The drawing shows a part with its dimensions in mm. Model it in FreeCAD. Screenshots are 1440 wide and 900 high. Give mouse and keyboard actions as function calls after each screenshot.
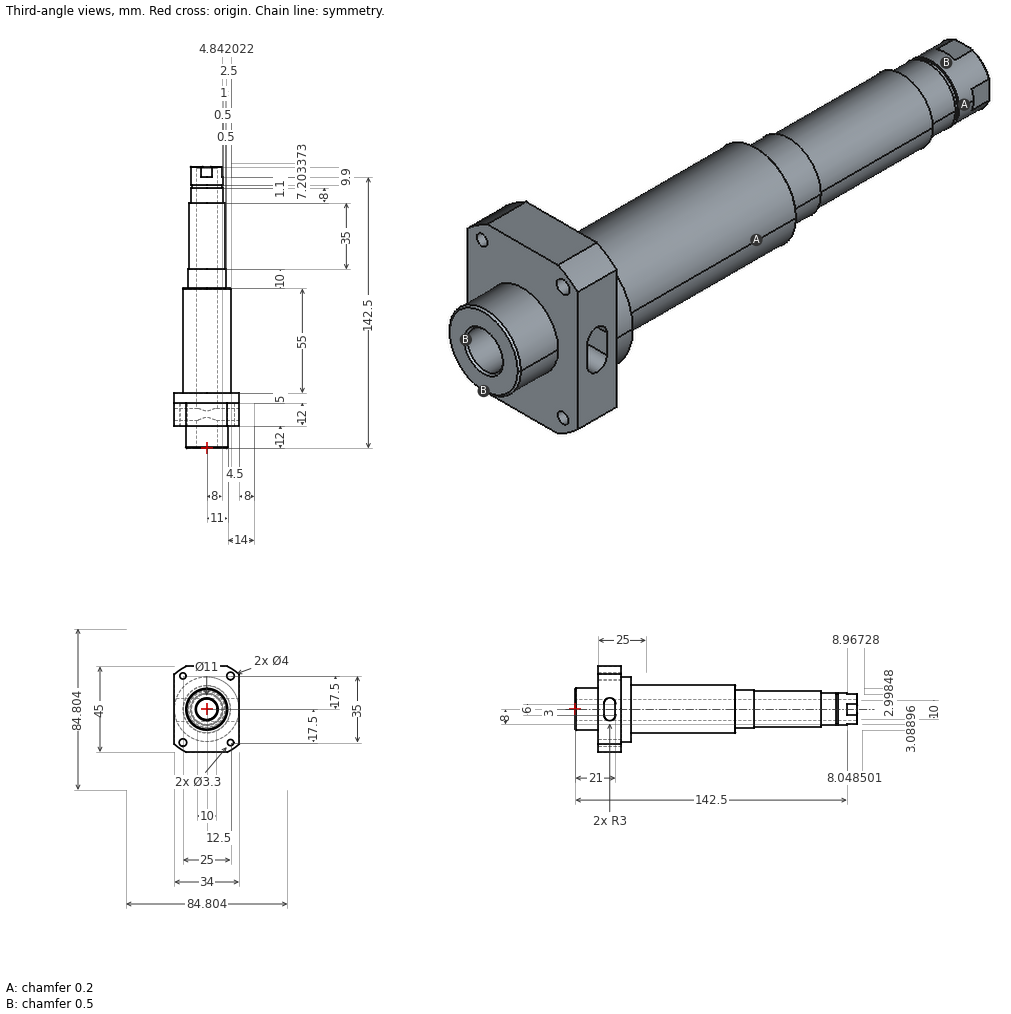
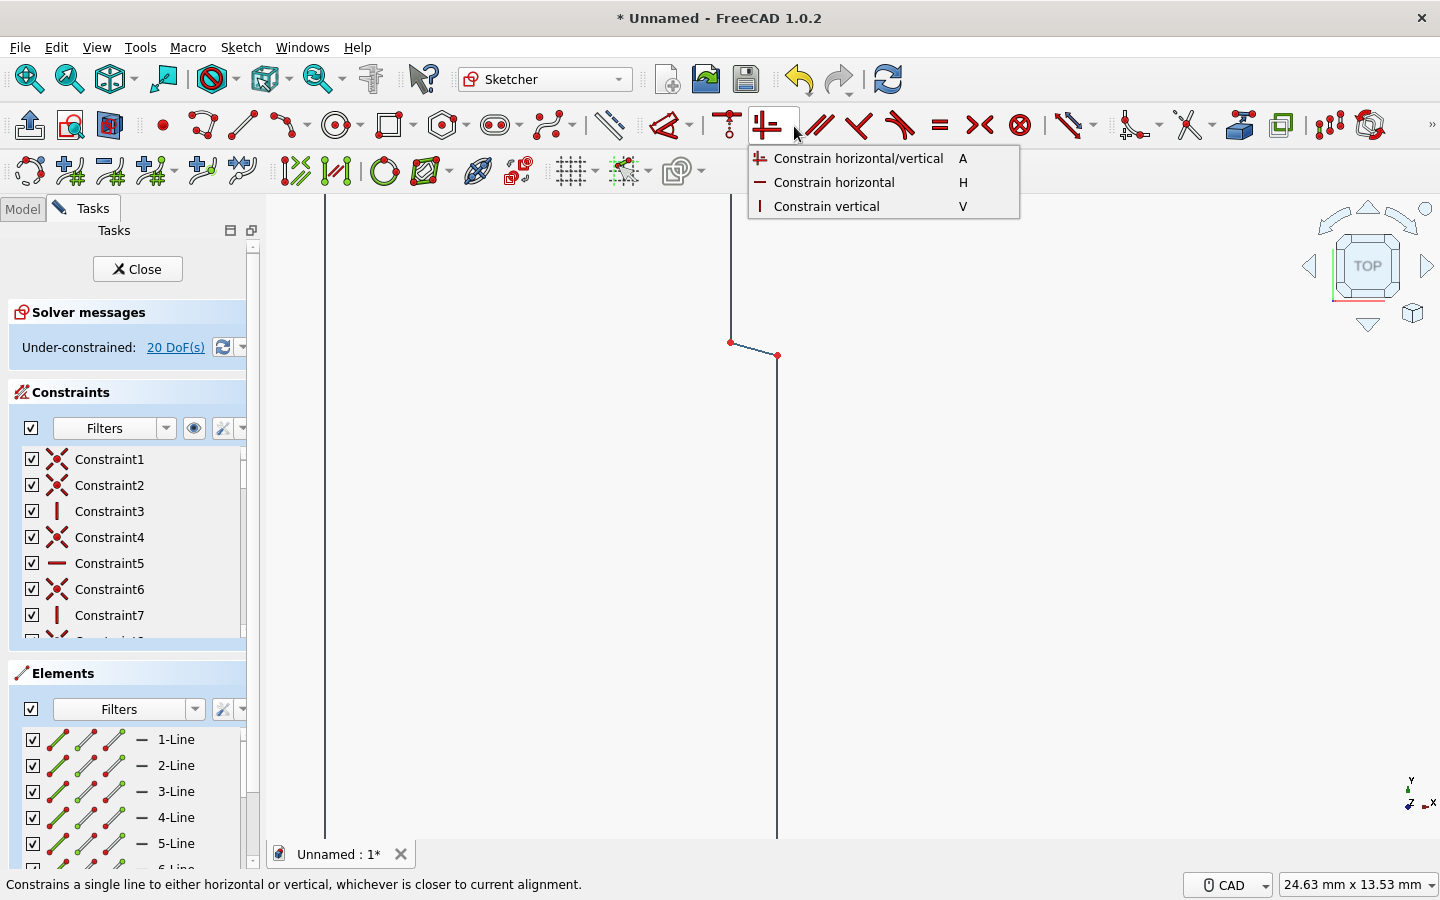
click(884, 182)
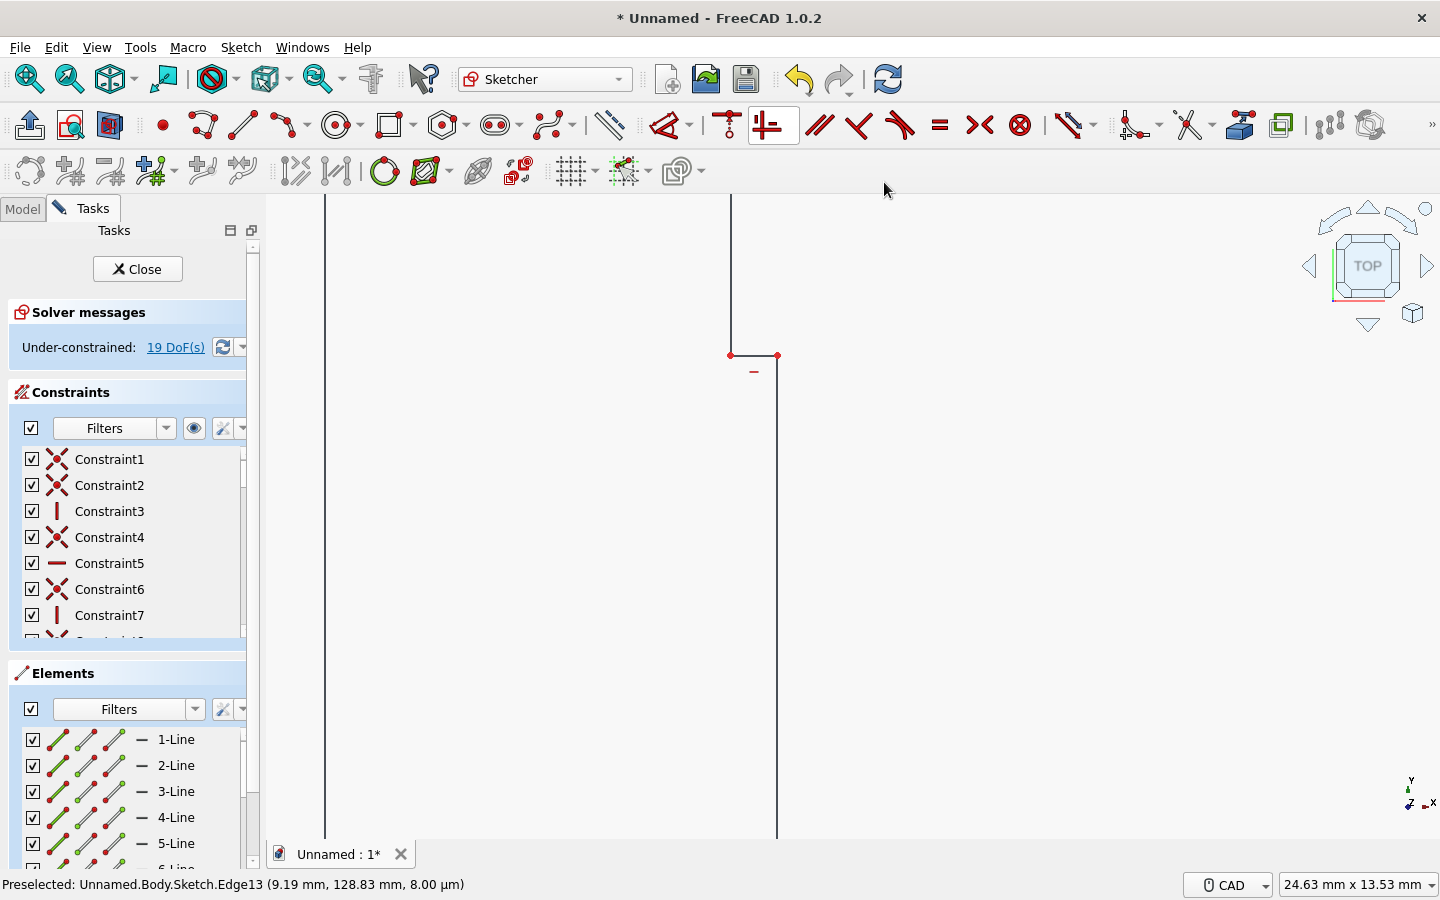
scroll(776, 358, down, 14)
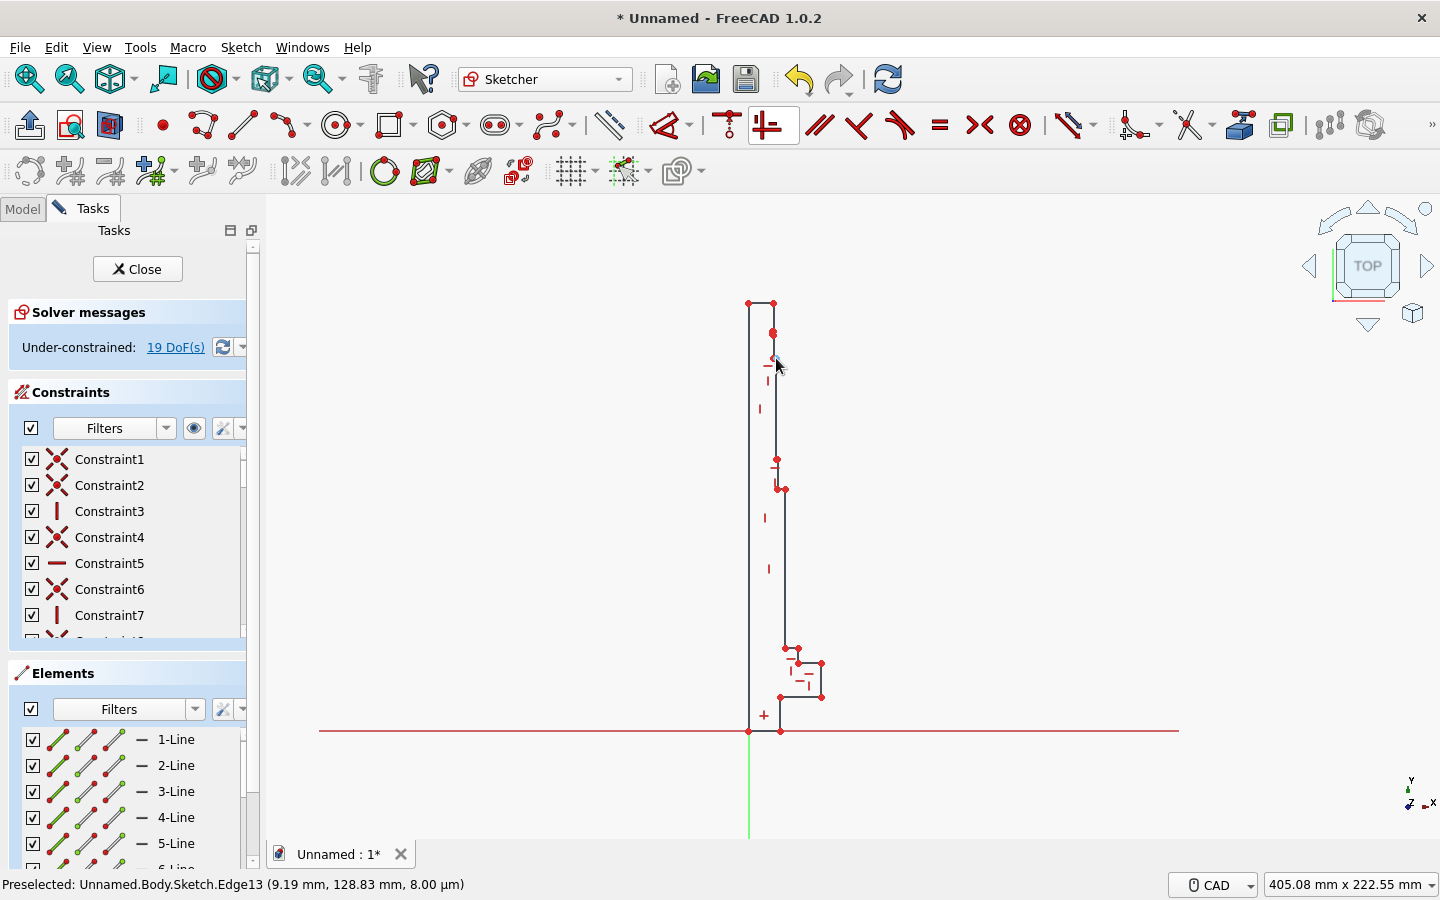
scroll(773, 335, up, 14)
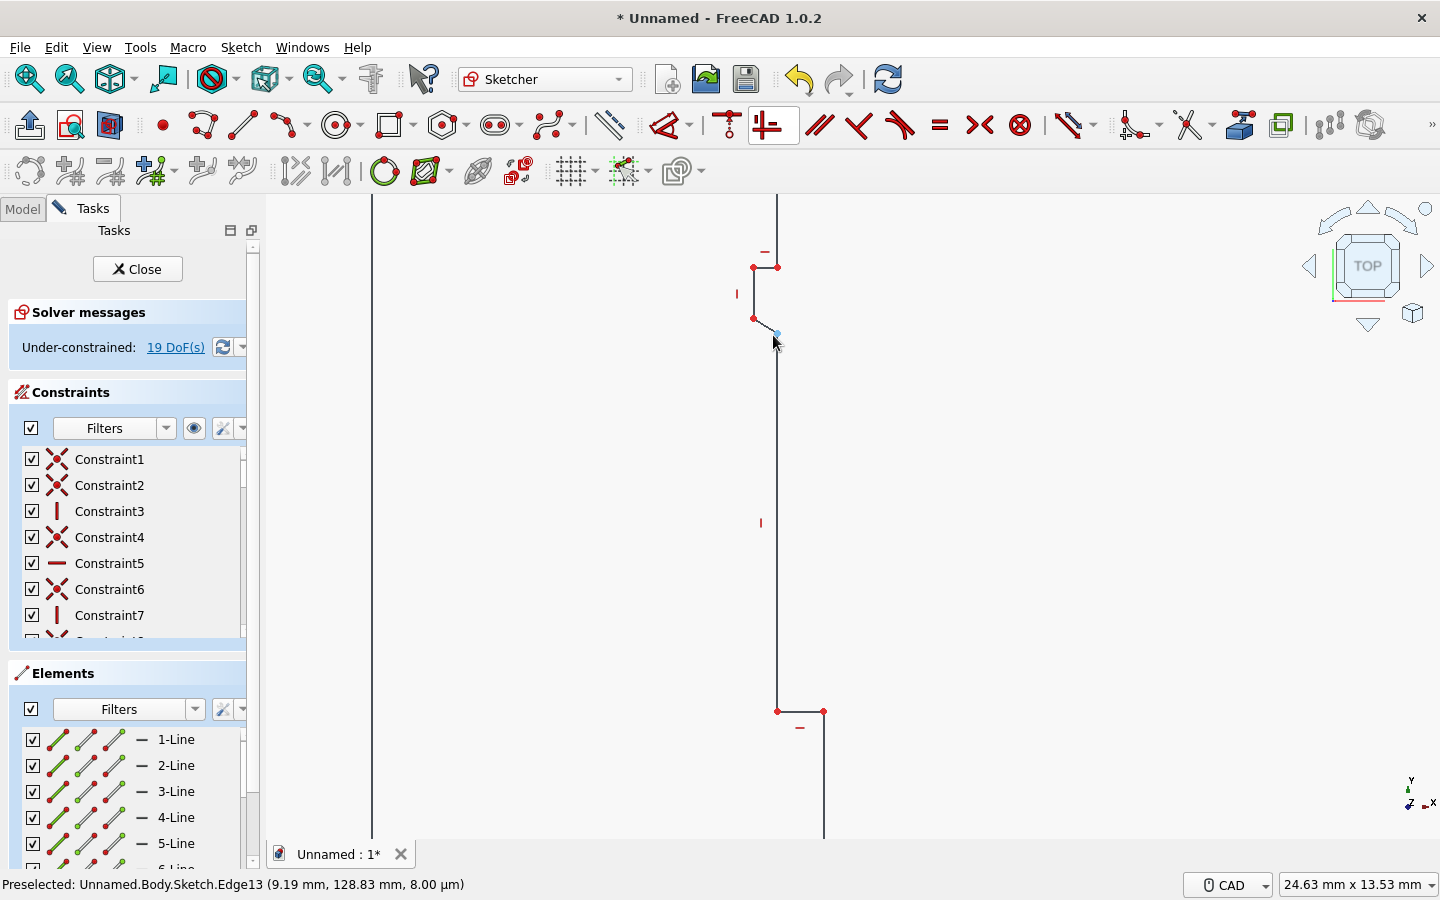
click(768, 328)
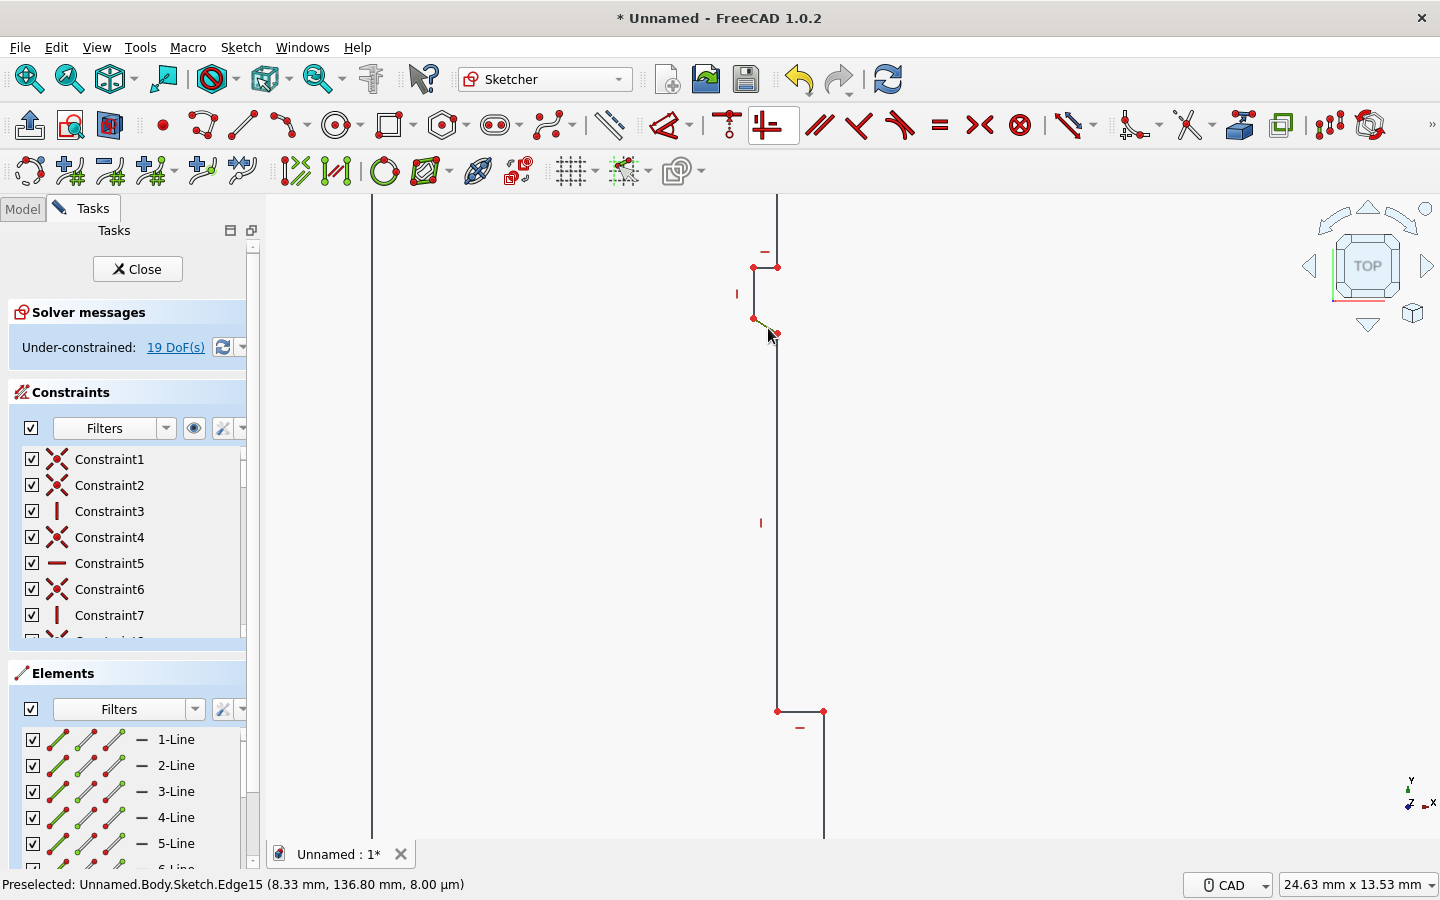
click(794, 126)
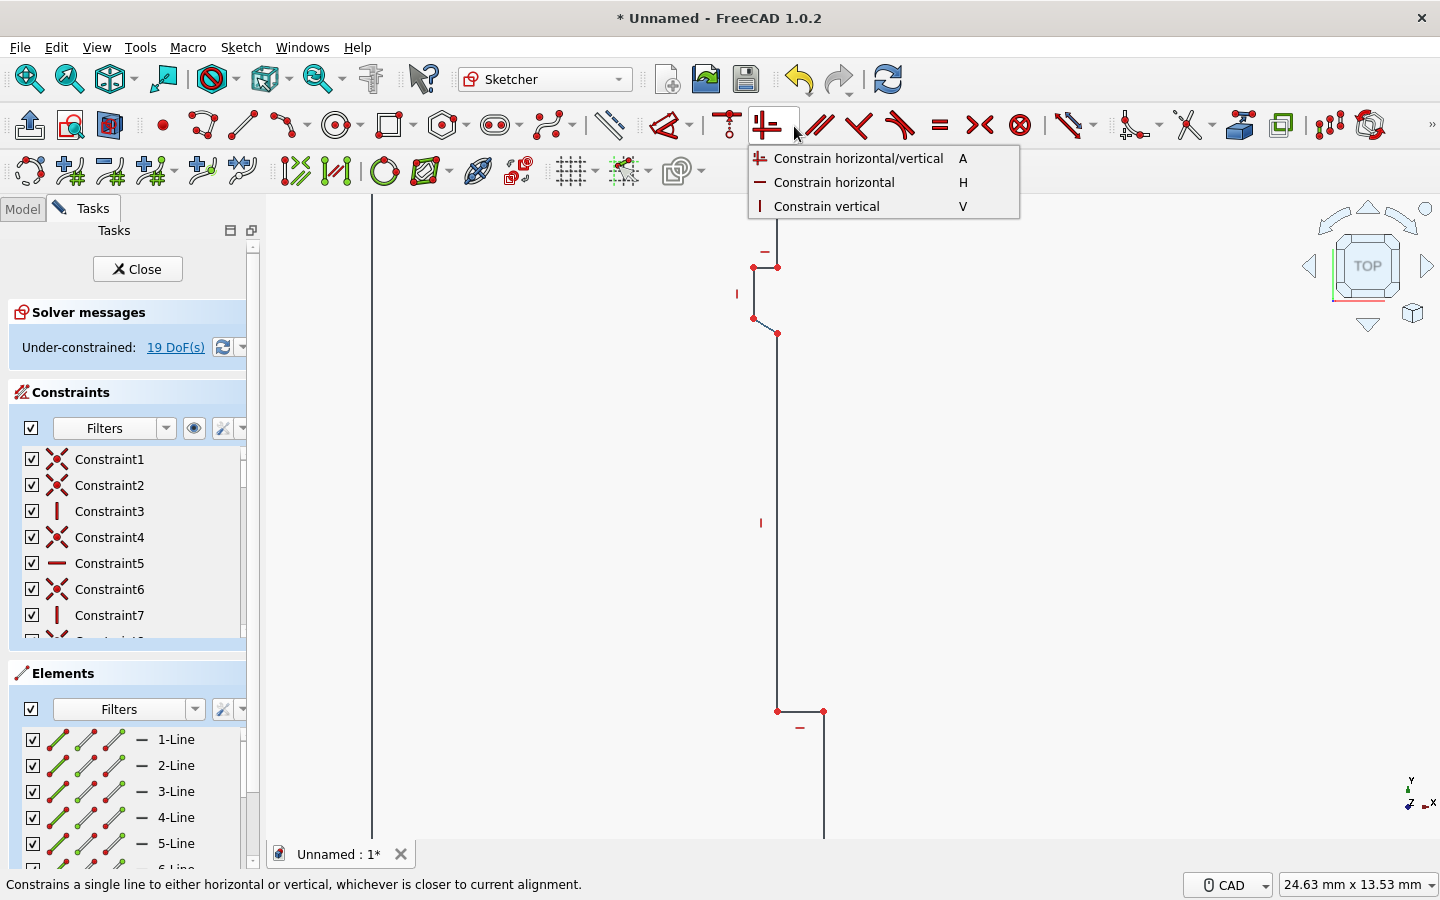
click(884, 182)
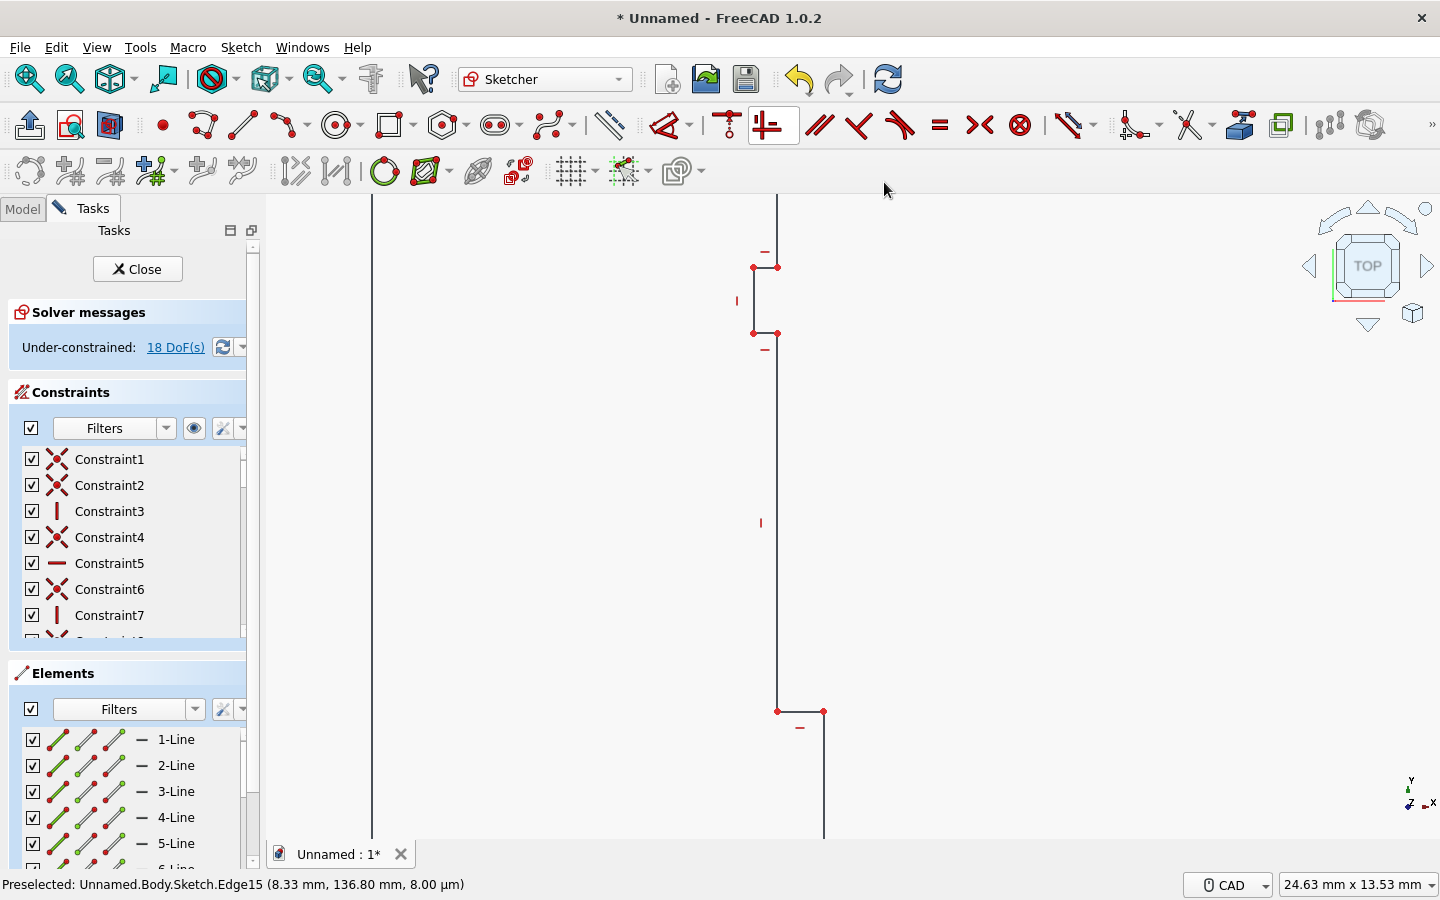
click(664, 126)